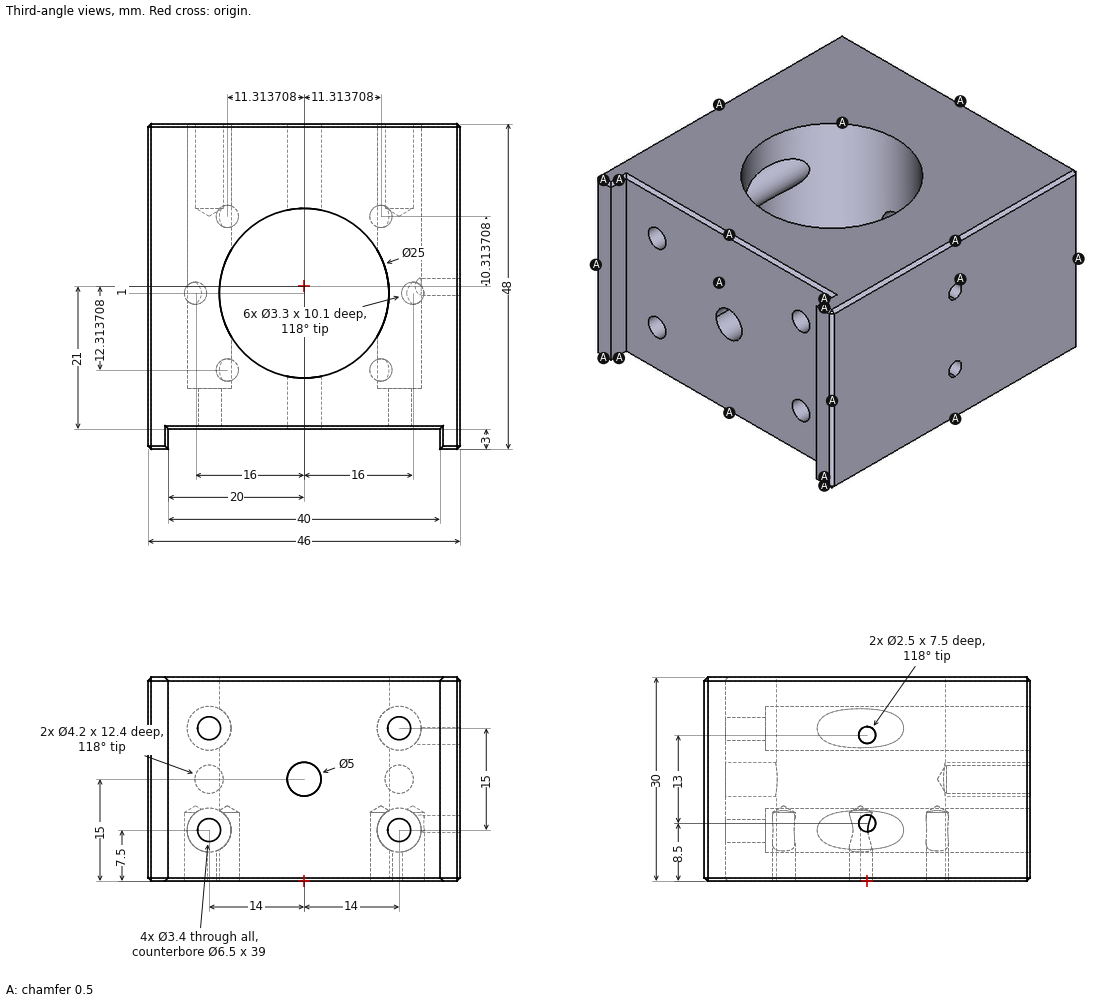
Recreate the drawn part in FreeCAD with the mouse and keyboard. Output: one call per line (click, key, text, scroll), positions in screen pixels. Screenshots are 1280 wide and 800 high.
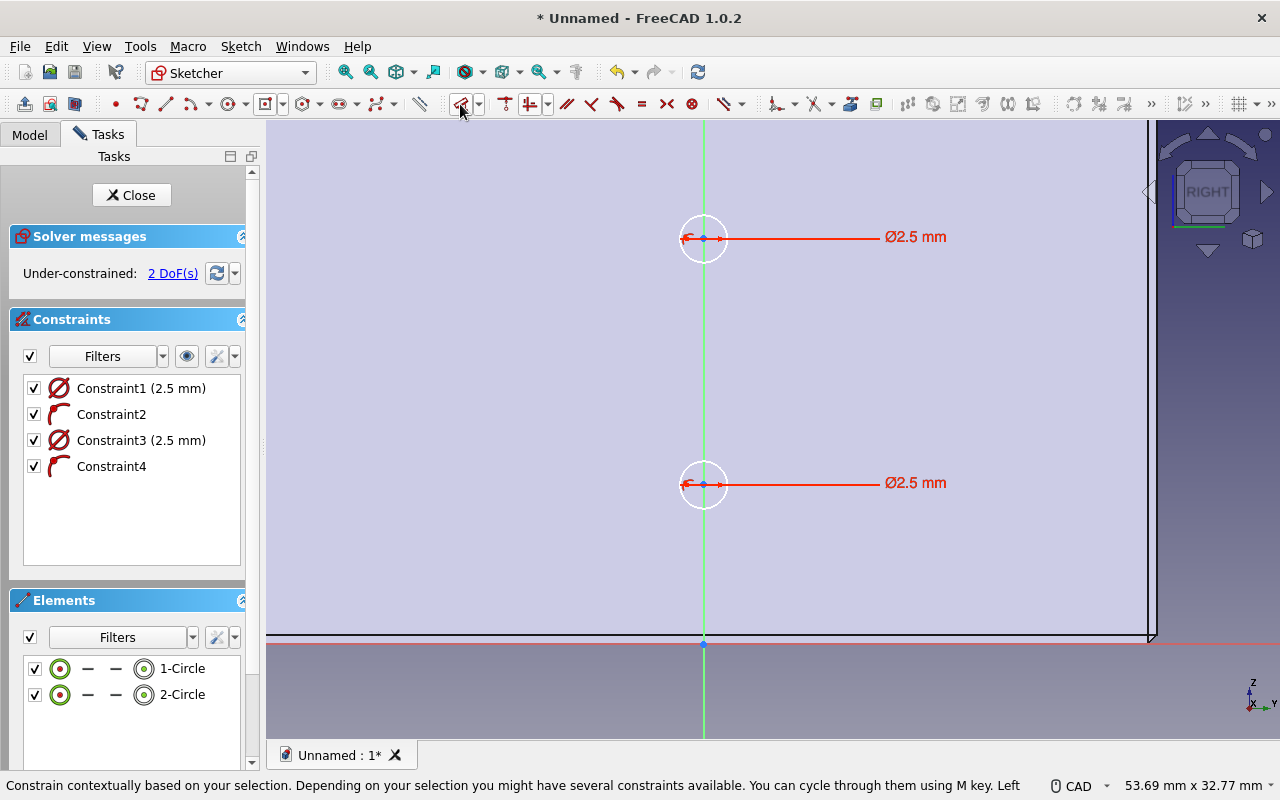
click(704, 485)
click(738, 565)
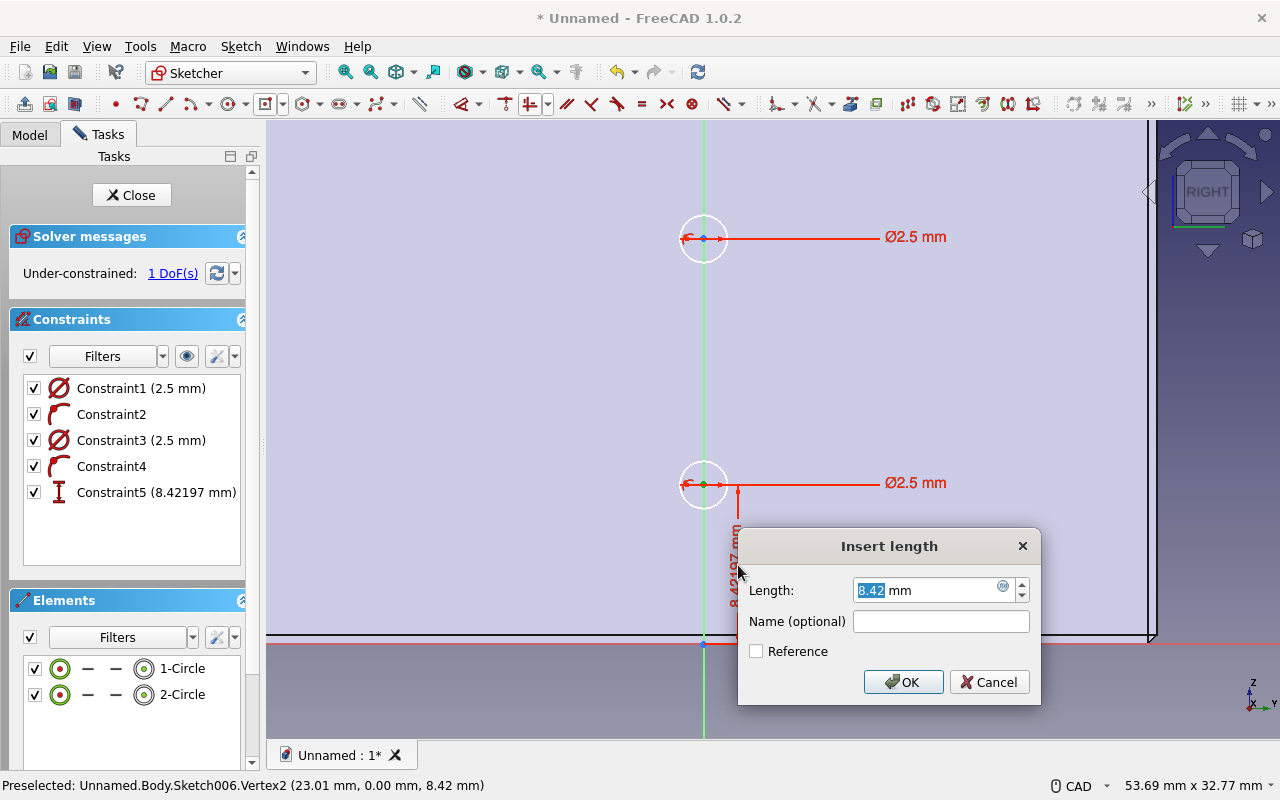
text(8.5)
key(Return)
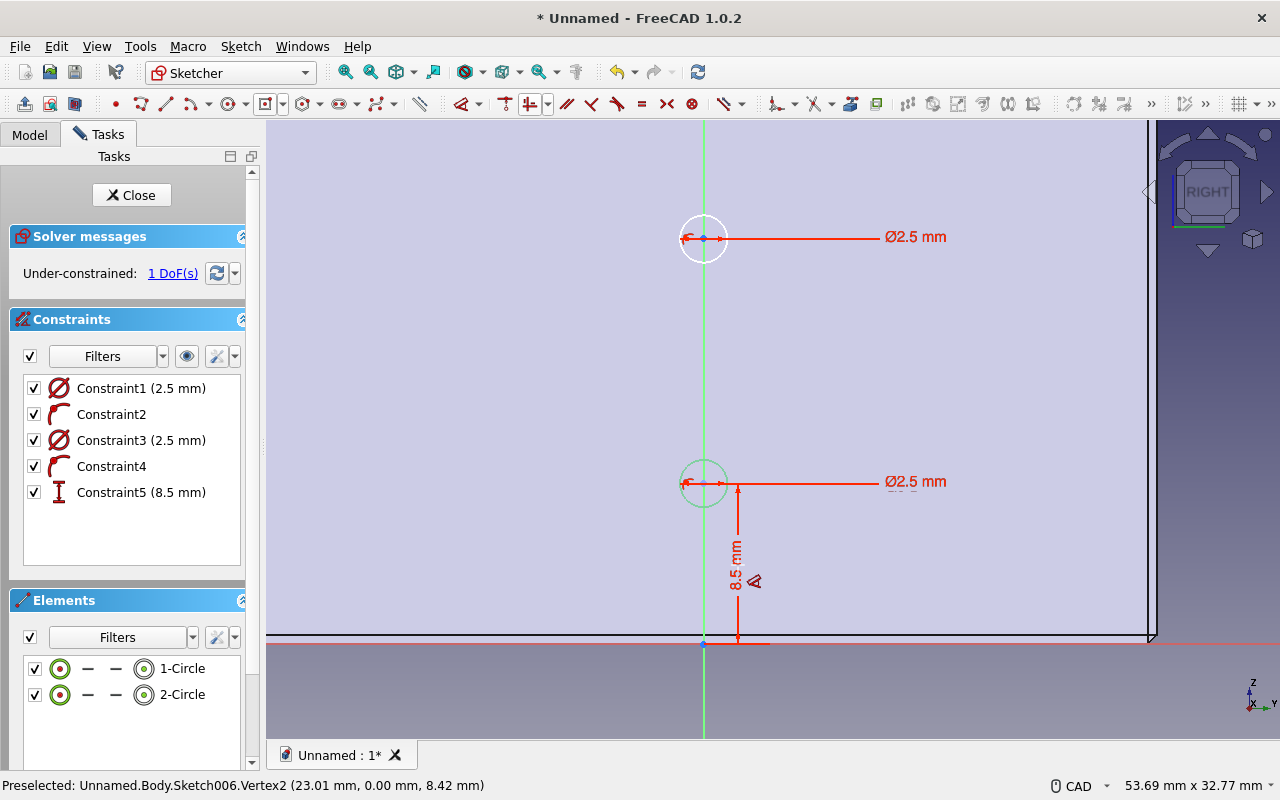
click(704, 239)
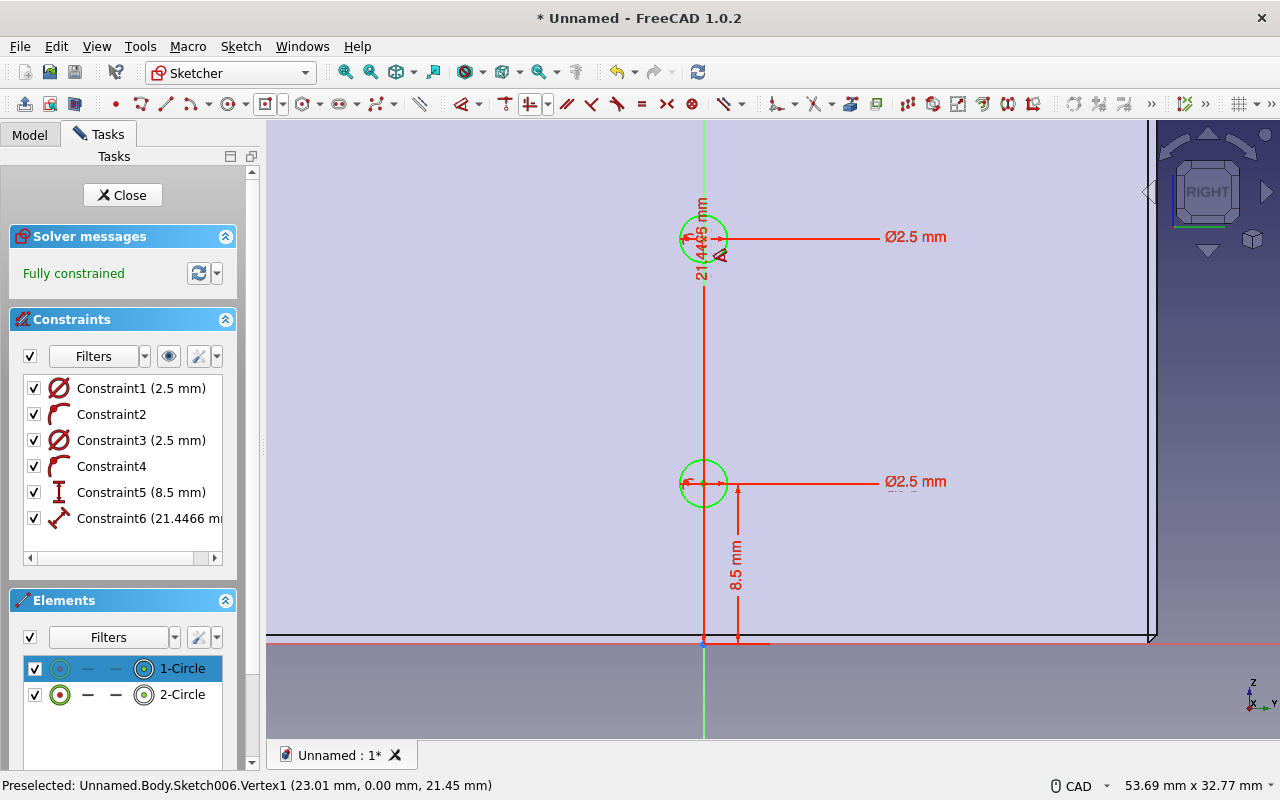
click(704, 484)
click(738, 361)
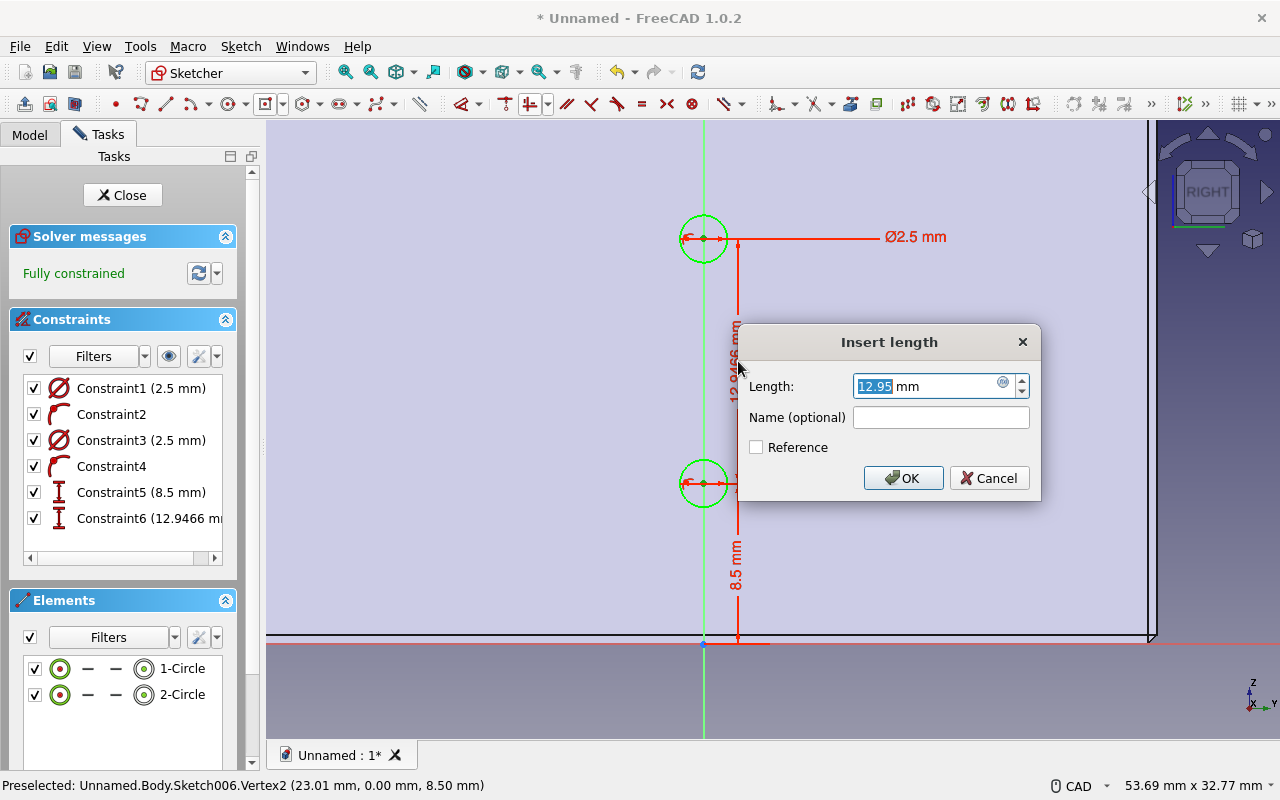
text(13)
key(Return)
key(Escape)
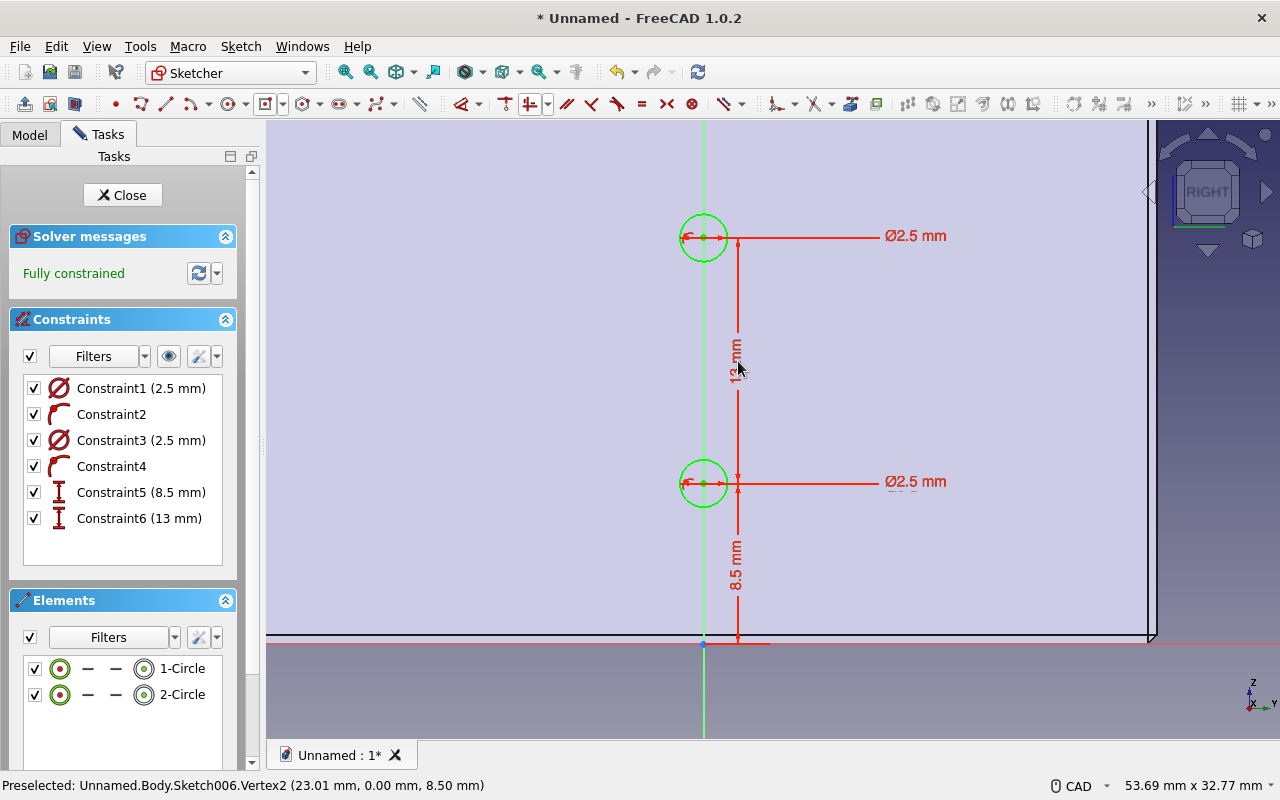
click(123, 195)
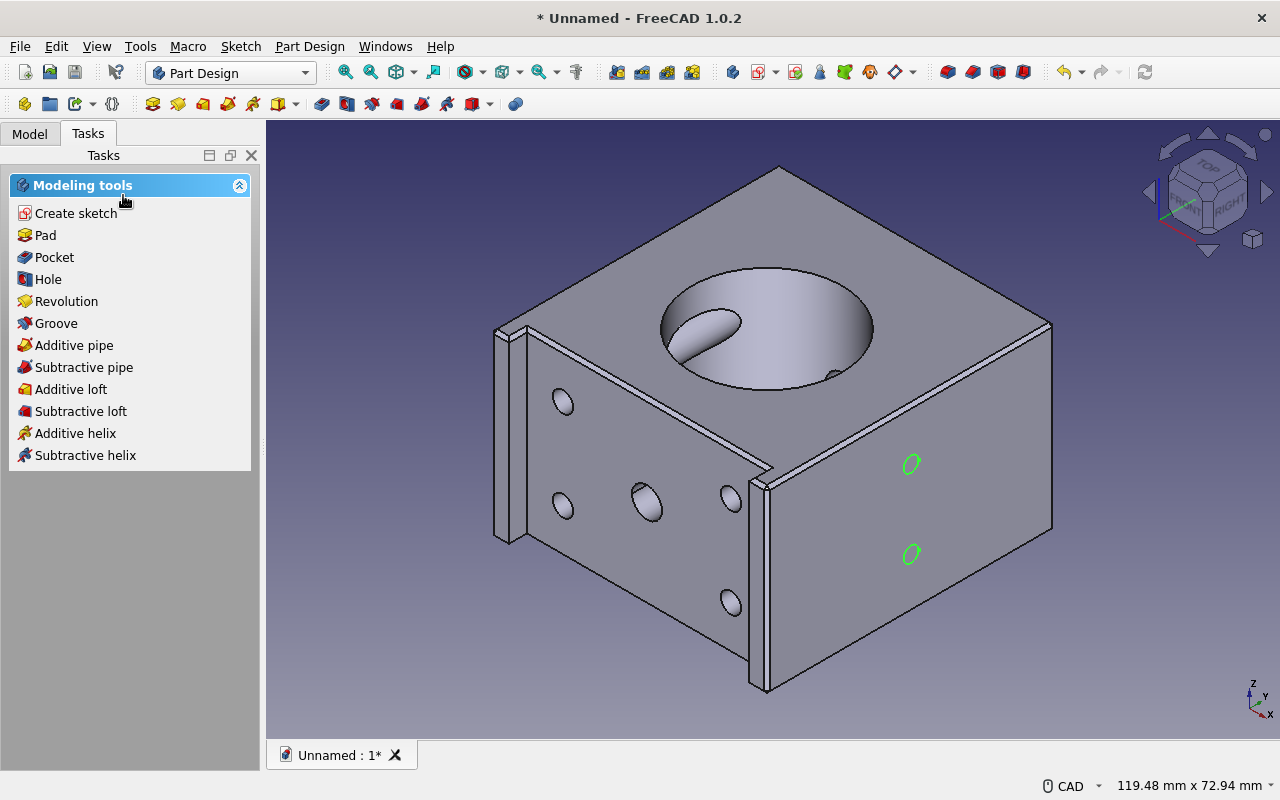
click(347, 104)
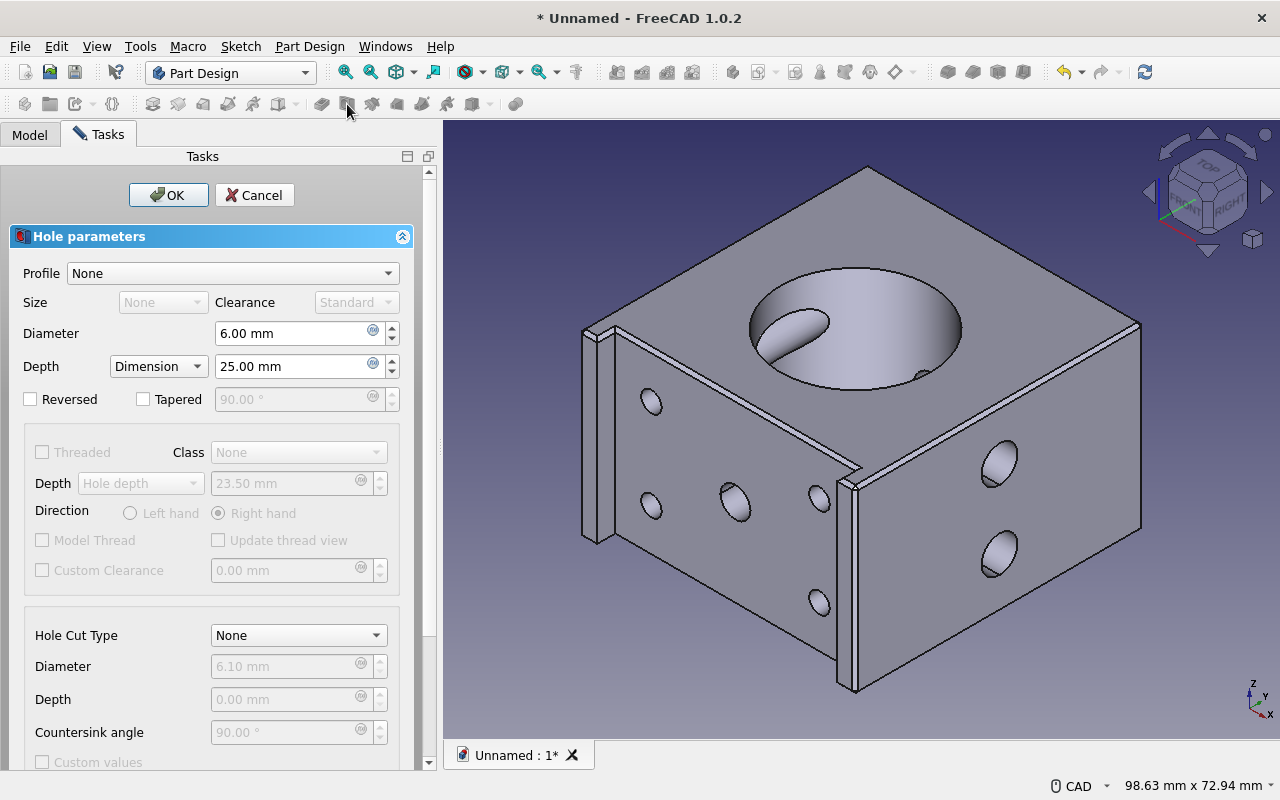
triple_click(300, 334)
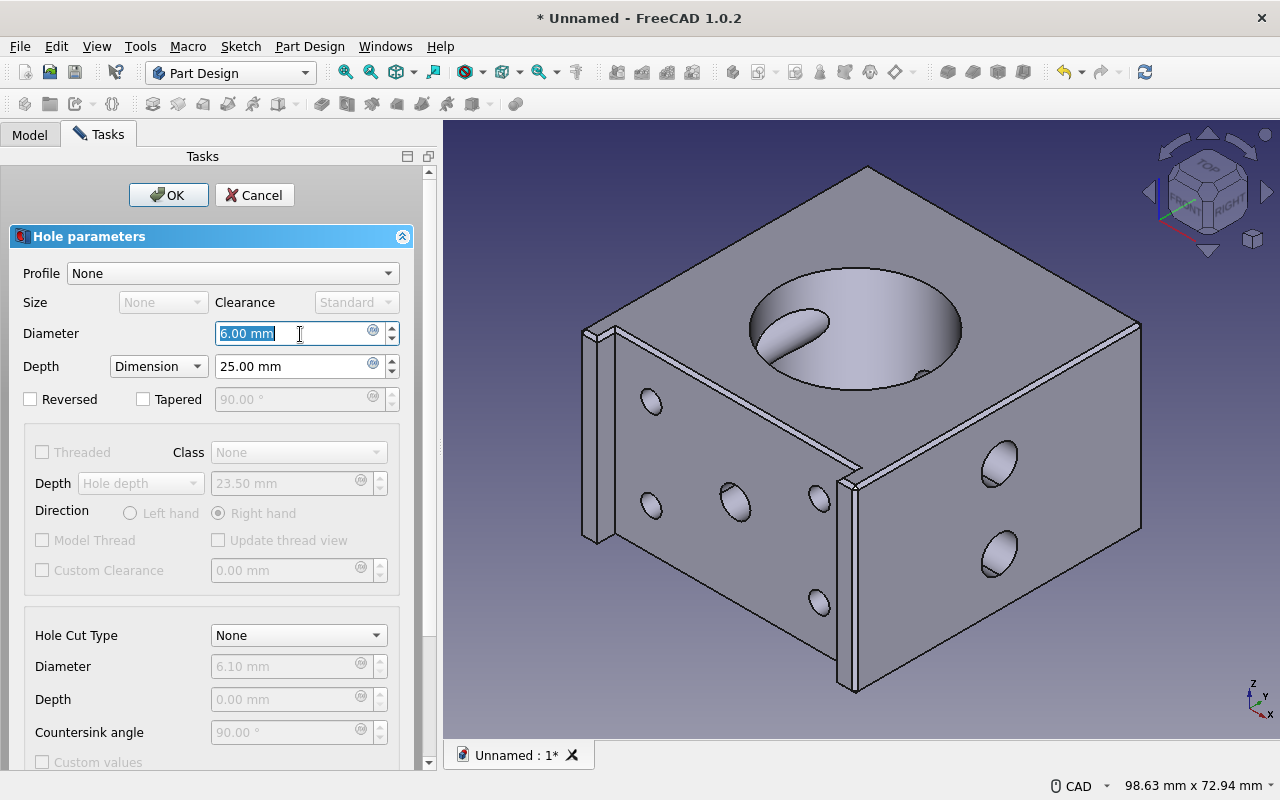
text(2.5)
key(Tab)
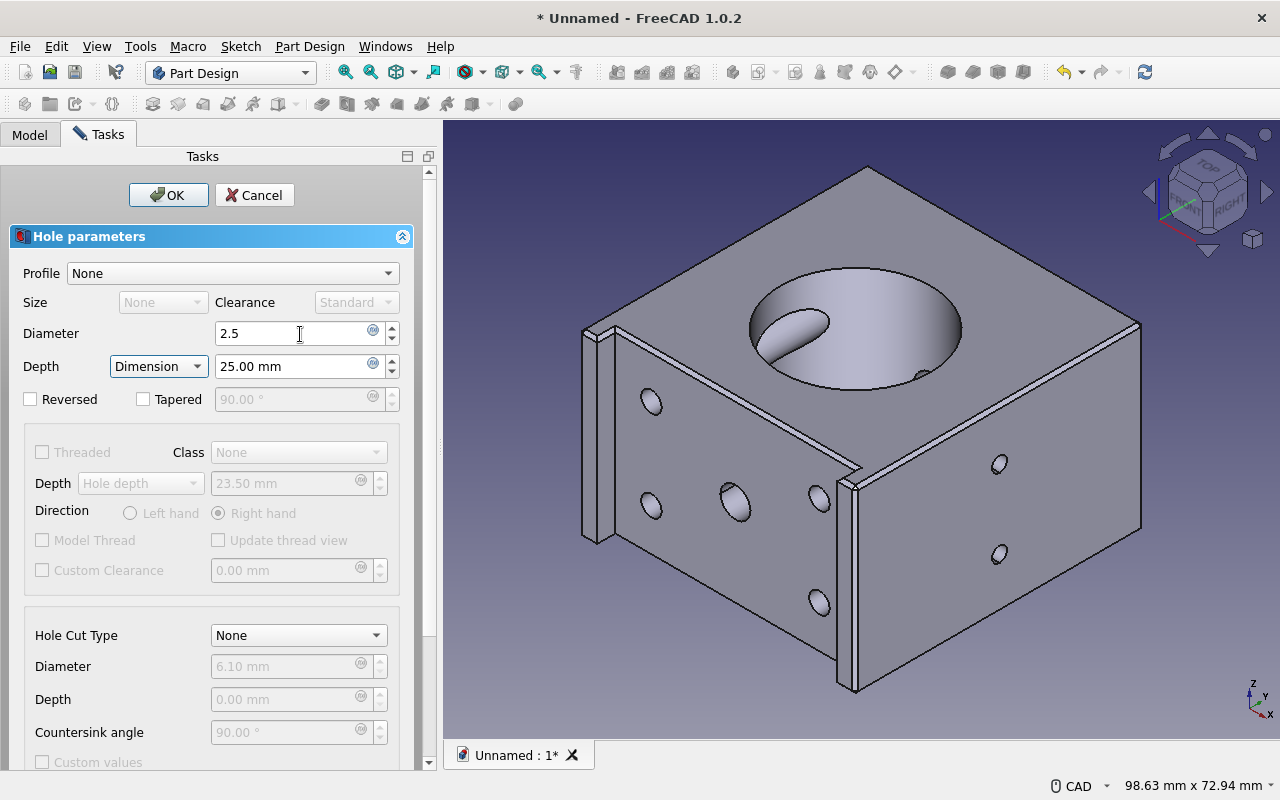
triple_click(300, 366)